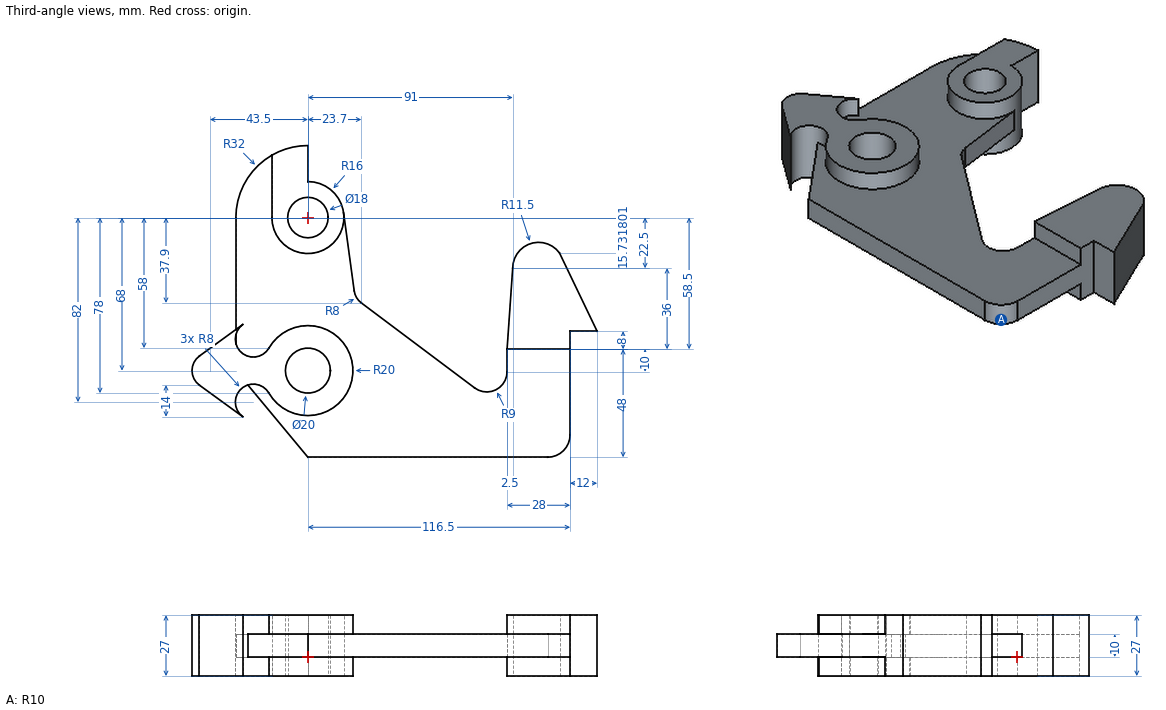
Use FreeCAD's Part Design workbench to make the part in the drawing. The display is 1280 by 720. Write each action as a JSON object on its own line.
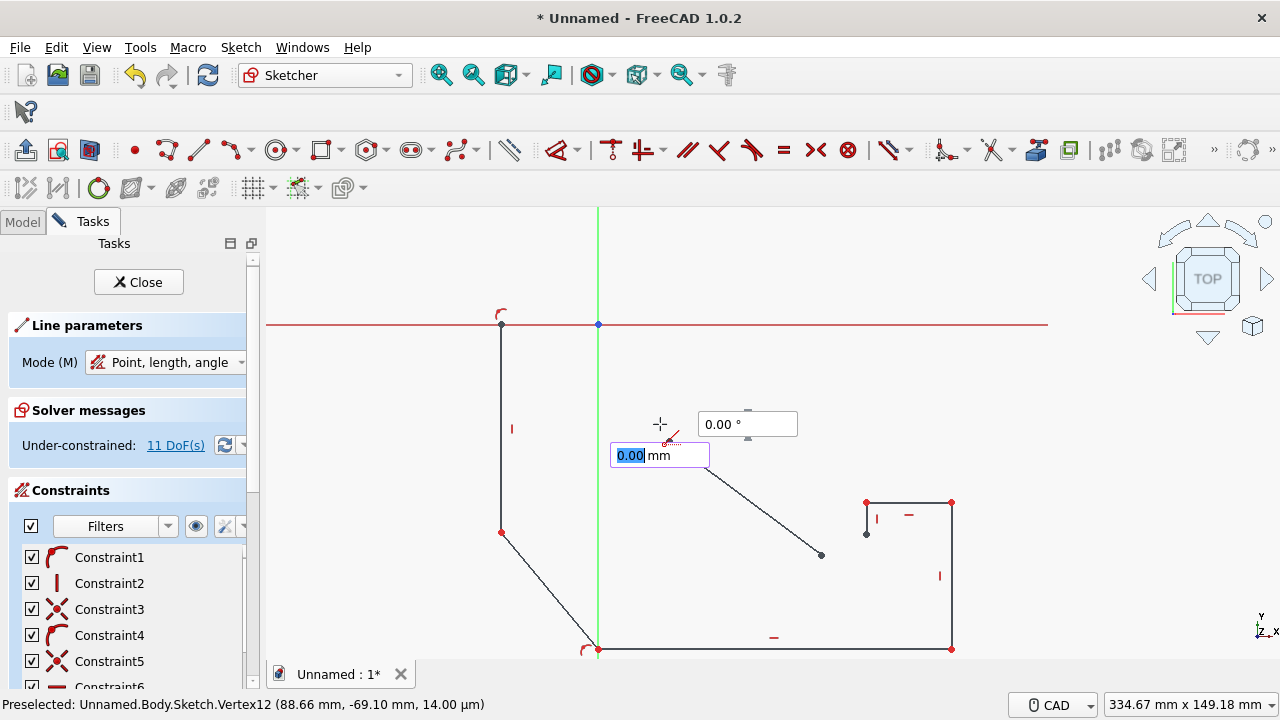
{"action": "scroll", "coordinate": [646, 318], "scroll_direction": "up", "scroll_amount": 5}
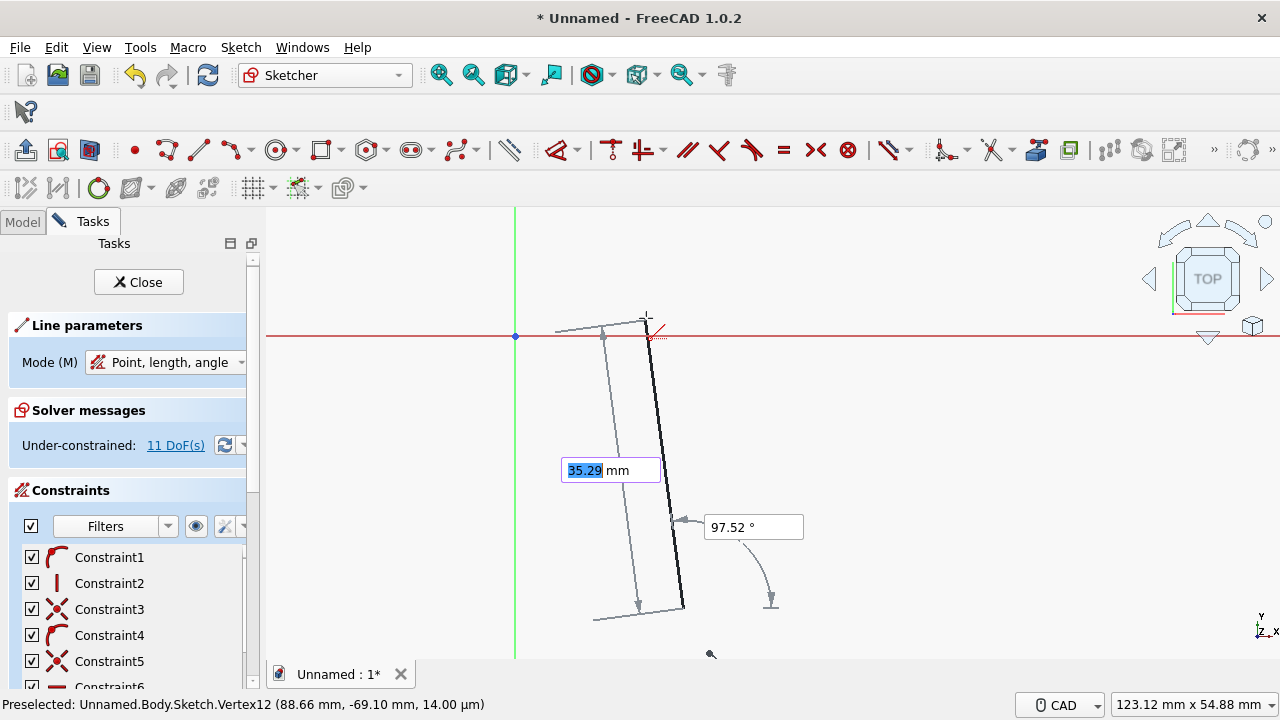
{"action": "left_click", "coordinate": [646, 318]}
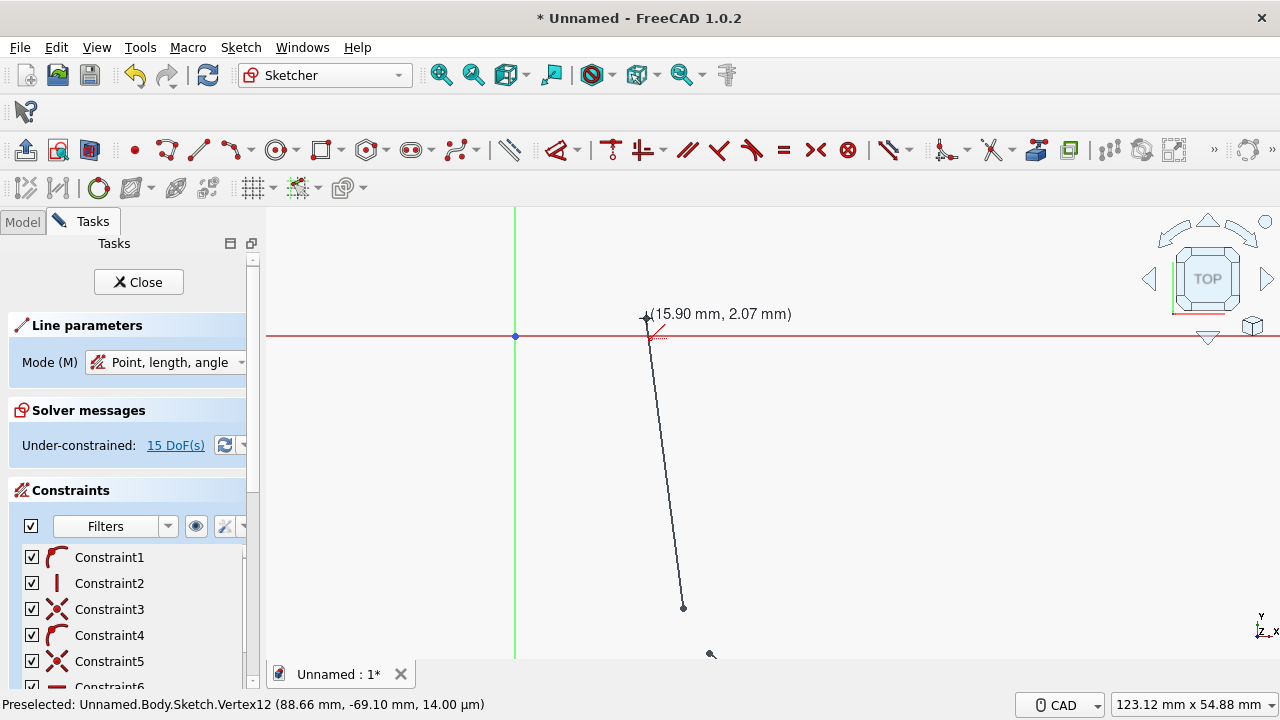
{"action": "scroll", "coordinate": [653, 364], "scroll_direction": "down", "scroll_amount": 7}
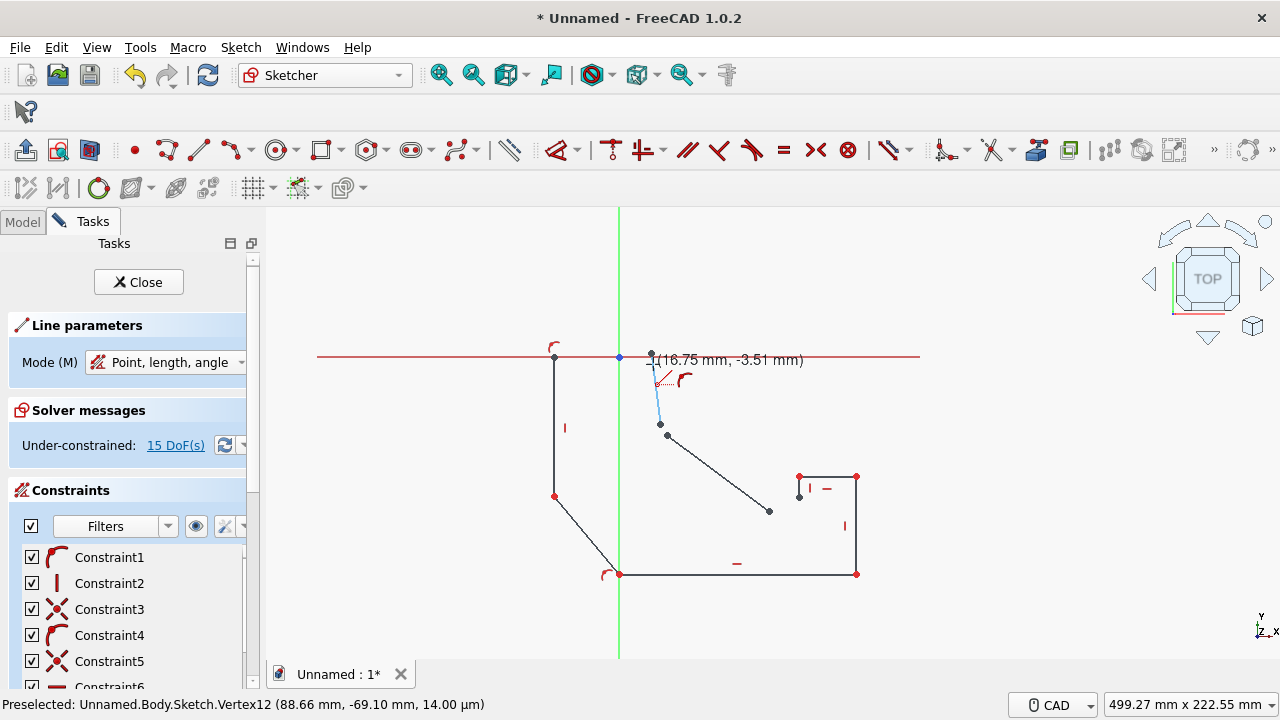
{"action": "left_click", "coordinate": [619, 325]}
{"action": "left_click", "coordinate": [628, 292]}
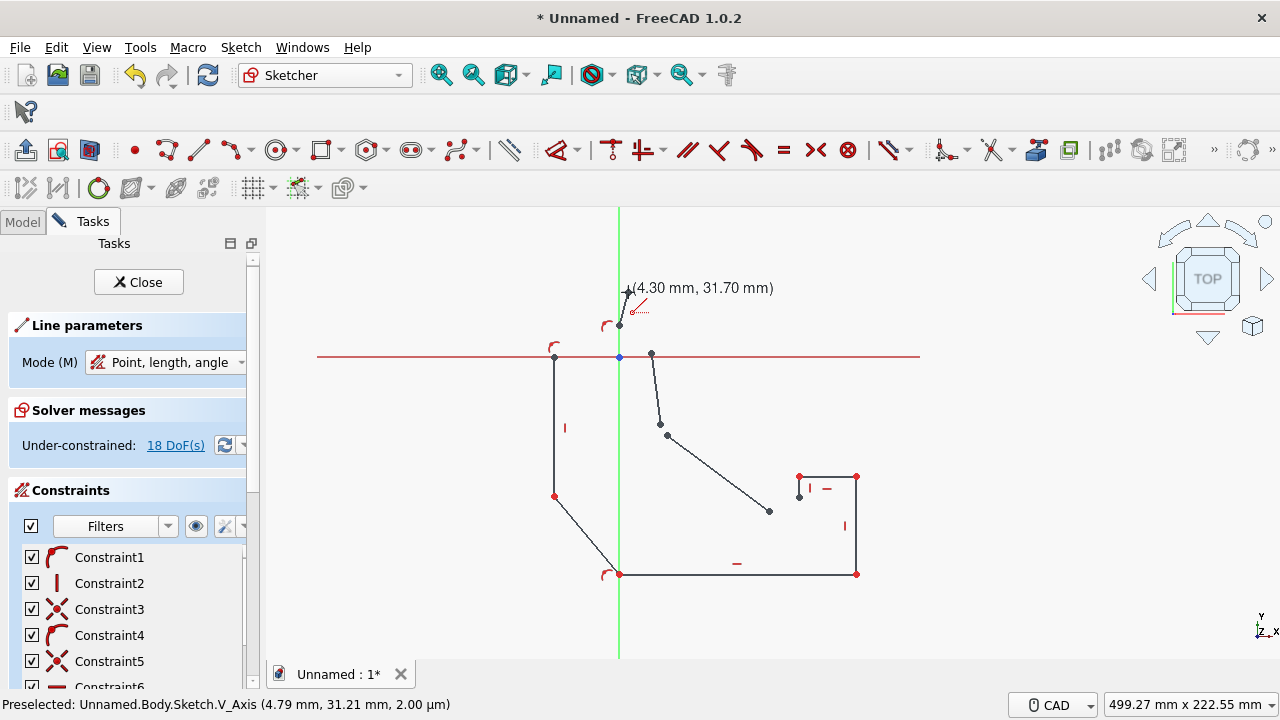
{"action": "left_click", "coordinate": [232, 150]}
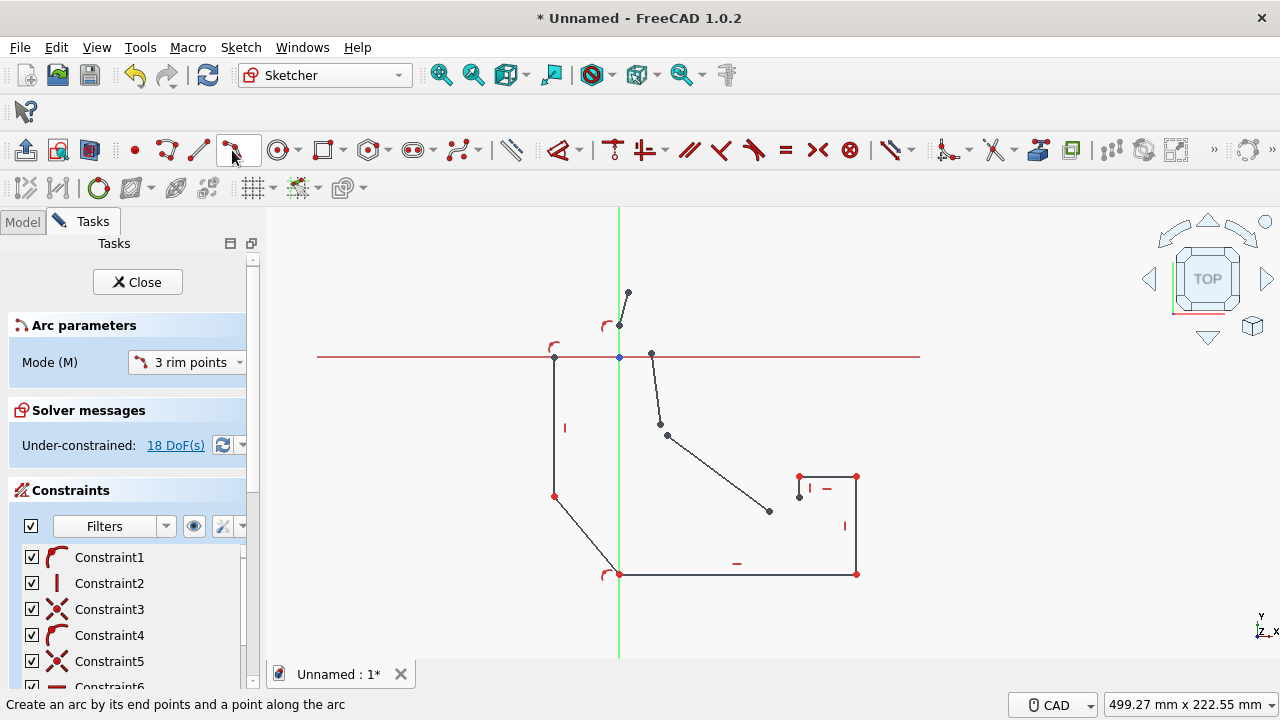
{"action": "scroll", "coordinate": [799, 496], "scroll_direction": "up", "scroll_amount": 3}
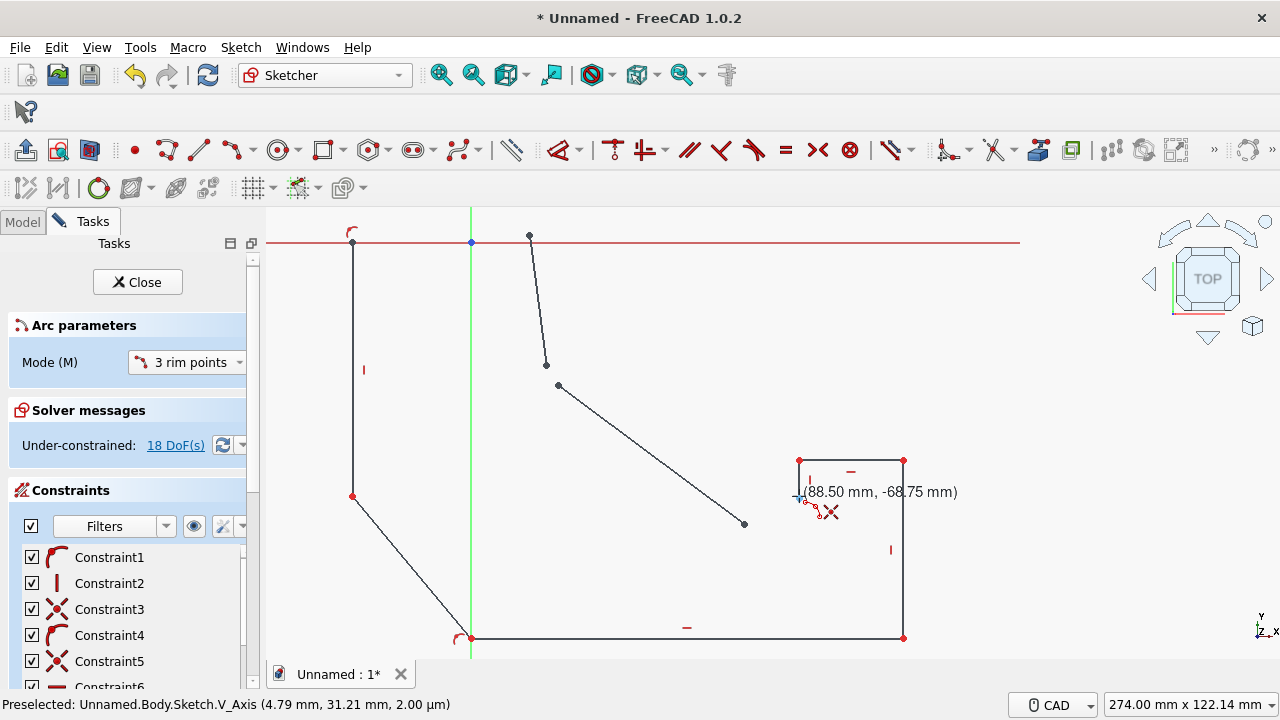
{"action": "left_click", "coordinate": [799, 499]}
{"action": "left_click", "coordinate": [745, 524]}
{"action": "left_click", "coordinate": [780, 526]}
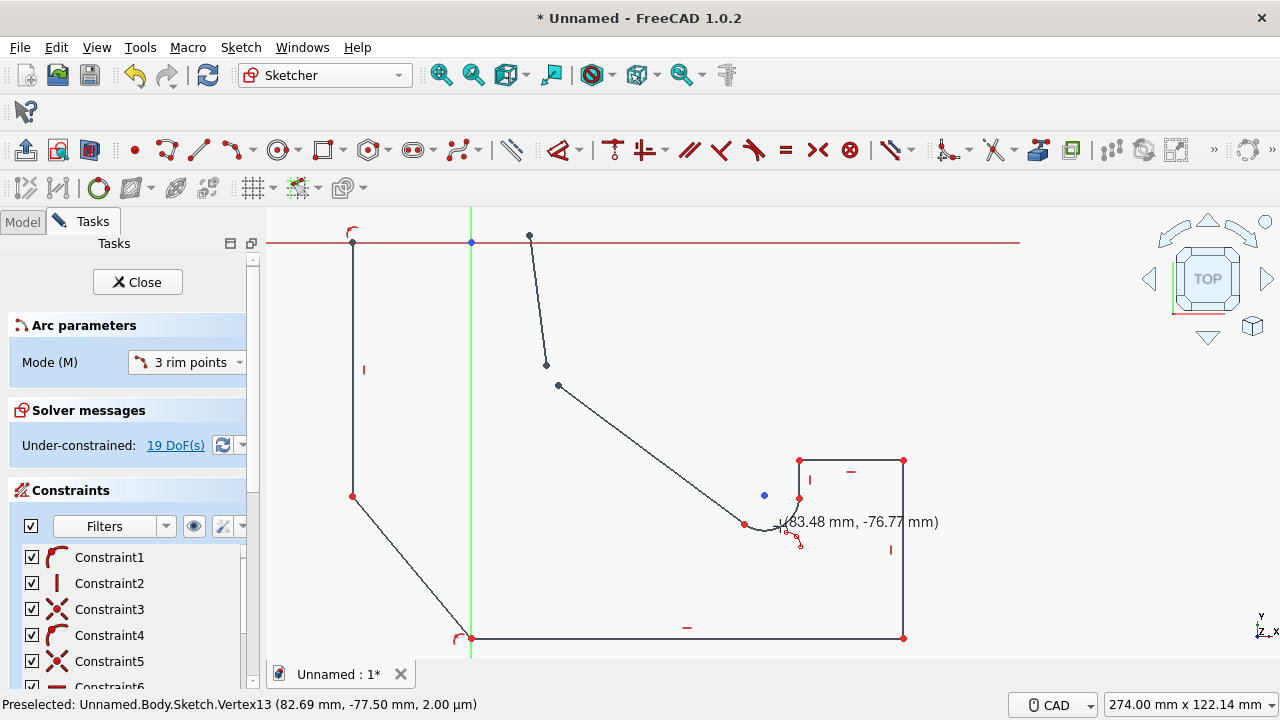
{"action": "left_click", "coordinate": [559, 386]}
{"action": "left_click", "coordinate": [547, 365]}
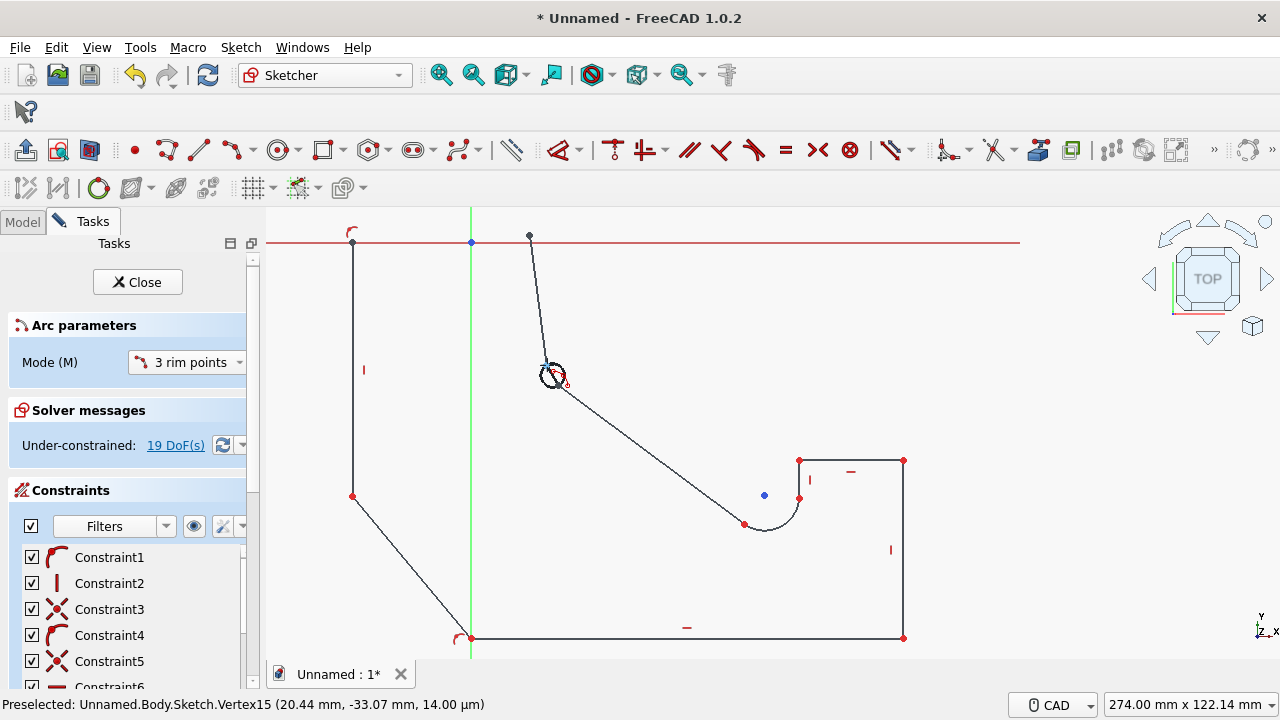
{"action": "scroll", "coordinate": [551, 374], "scroll_direction": "up", "scroll_amount": 10}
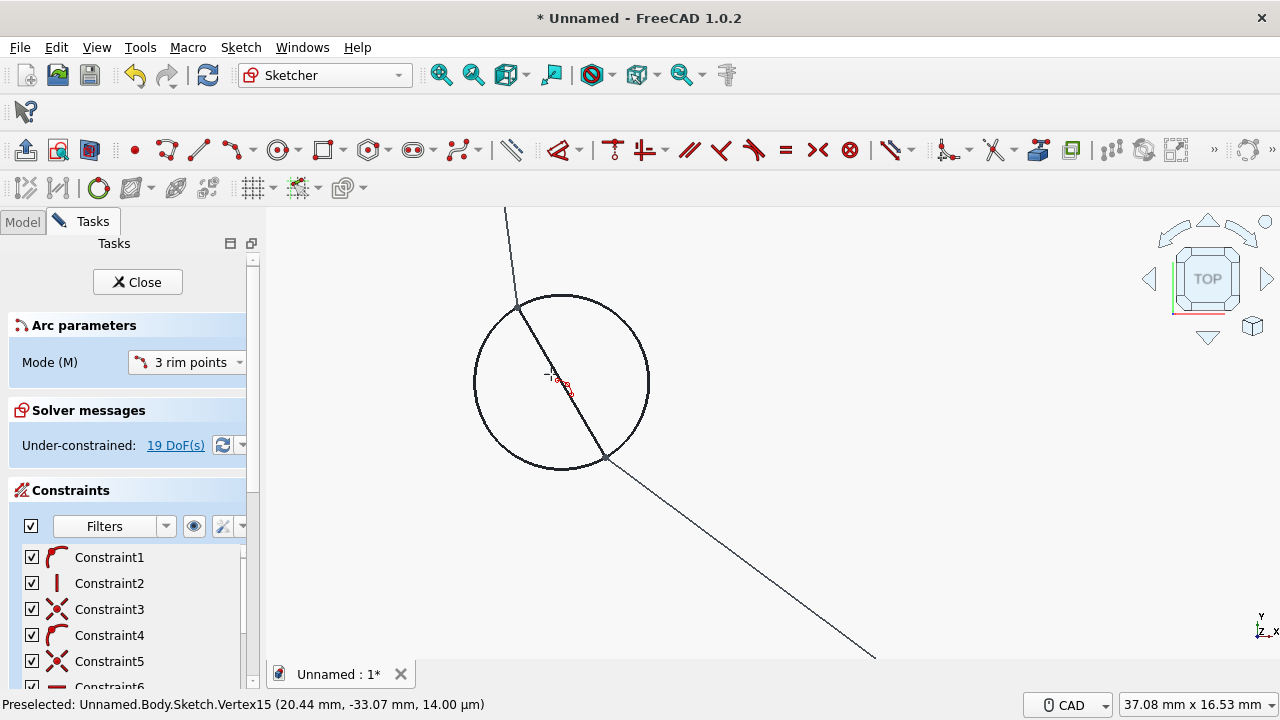
{"action": "left_click", "coordinate": [549, 375]}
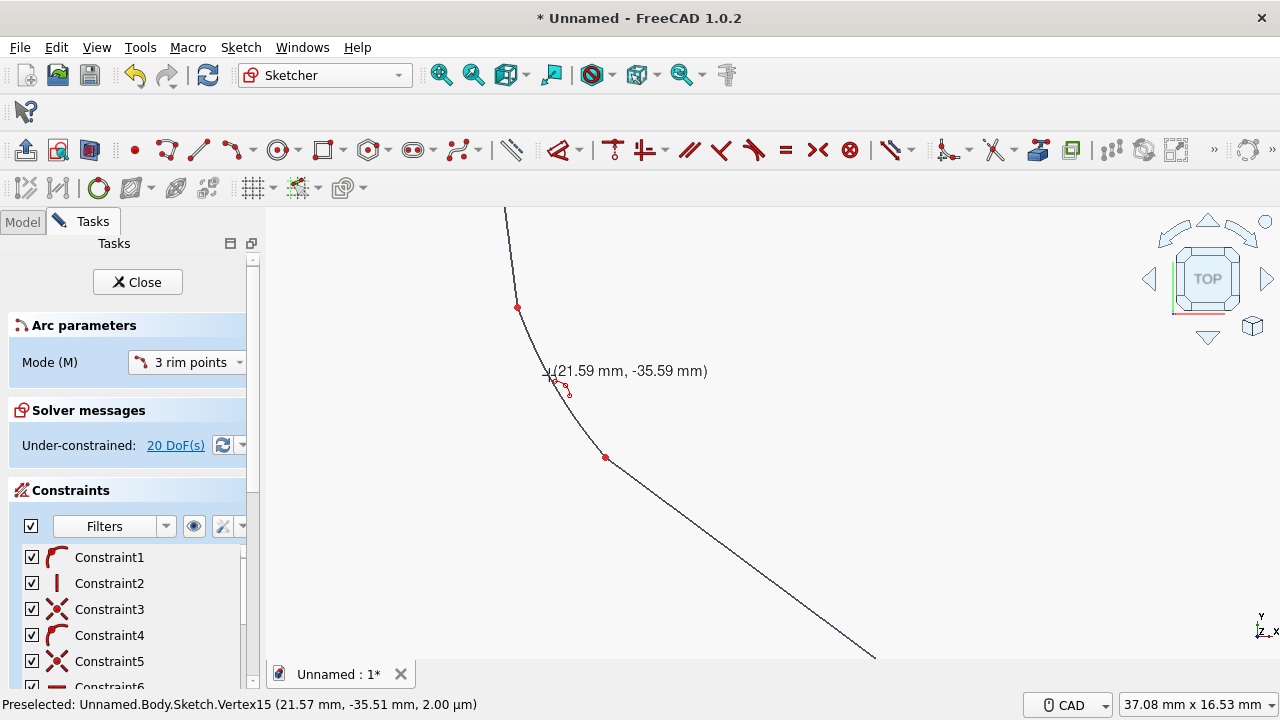
{"action": "scroll", "coordinate": [672, 434], "scroll_direction": "down", "scroll_amount": 13}